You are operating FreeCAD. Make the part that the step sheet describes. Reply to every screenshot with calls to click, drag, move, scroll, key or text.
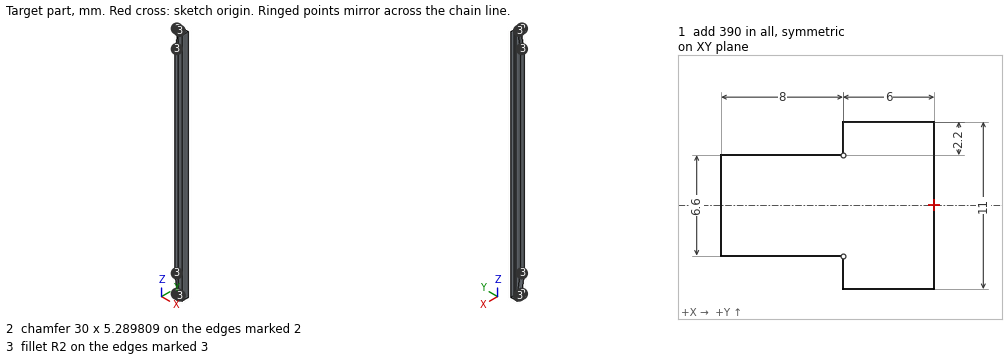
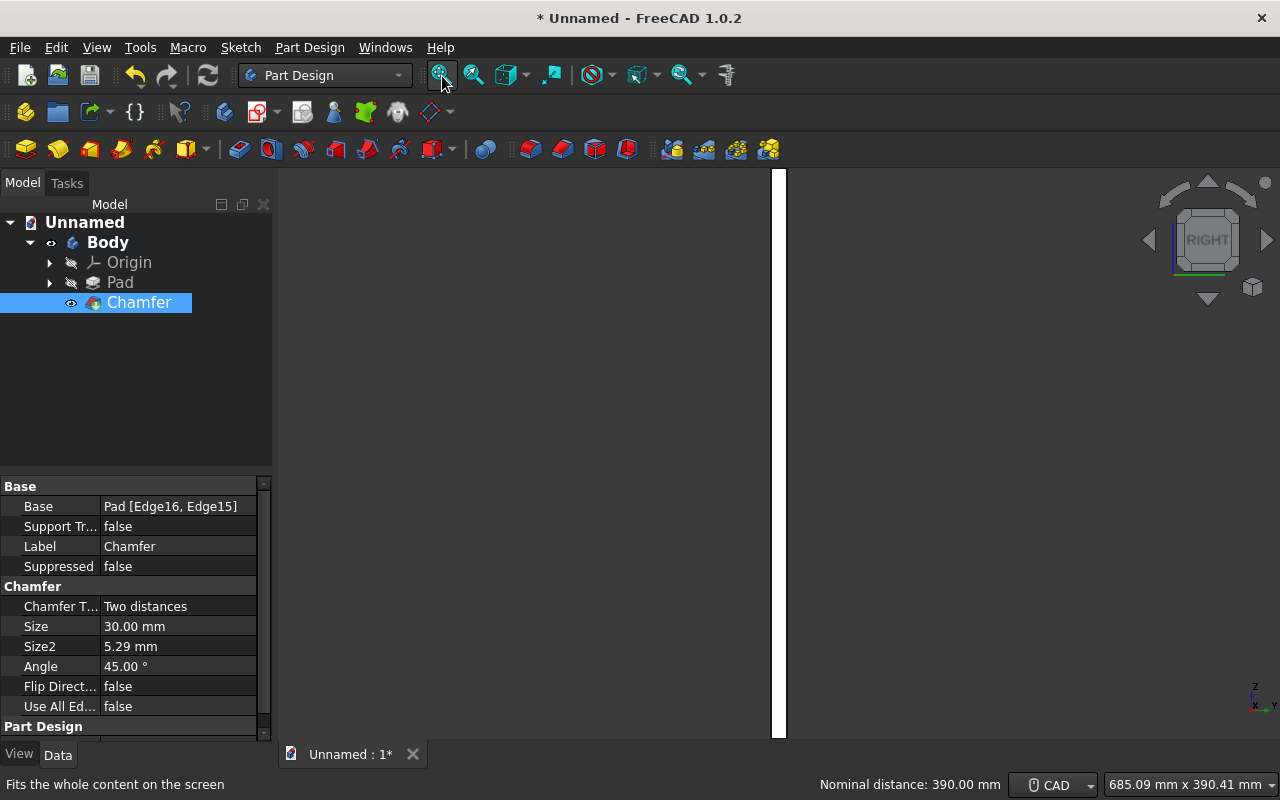
click(442, 76)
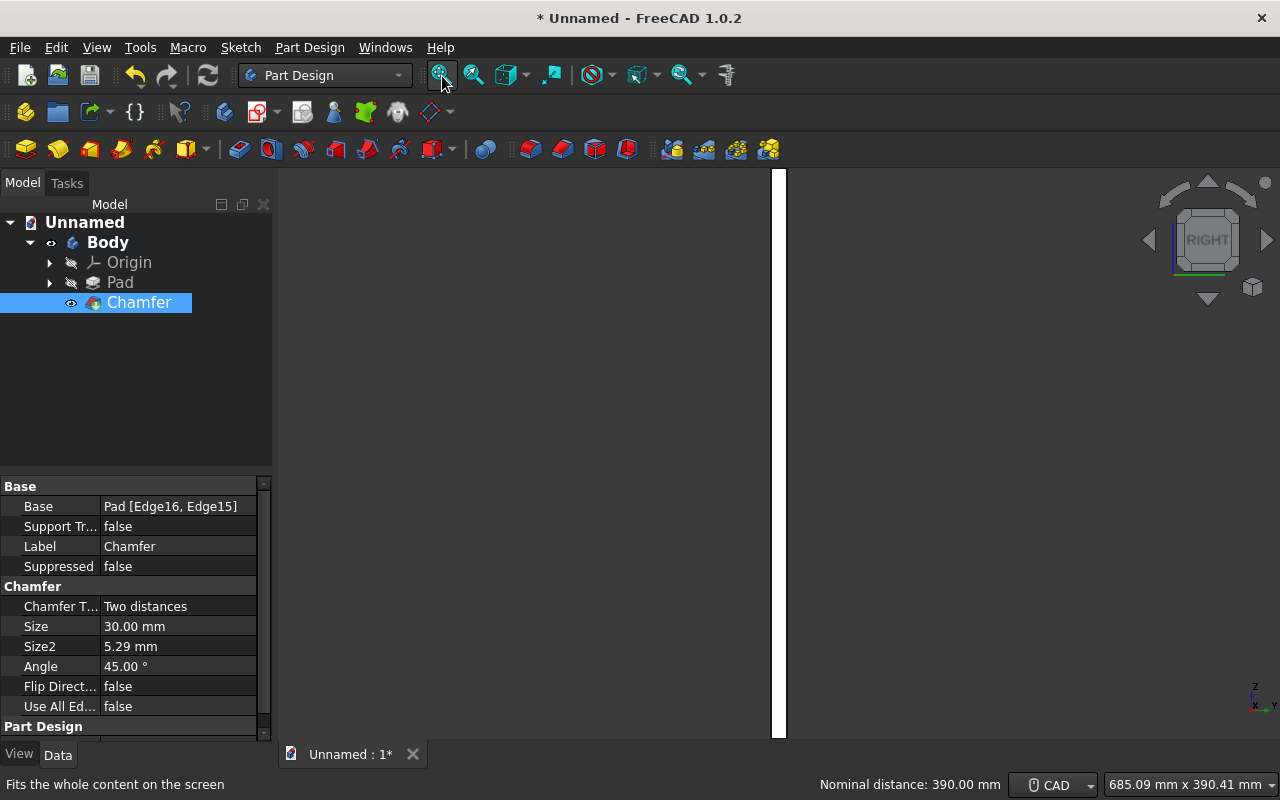
scroll(779, 211, up, 8)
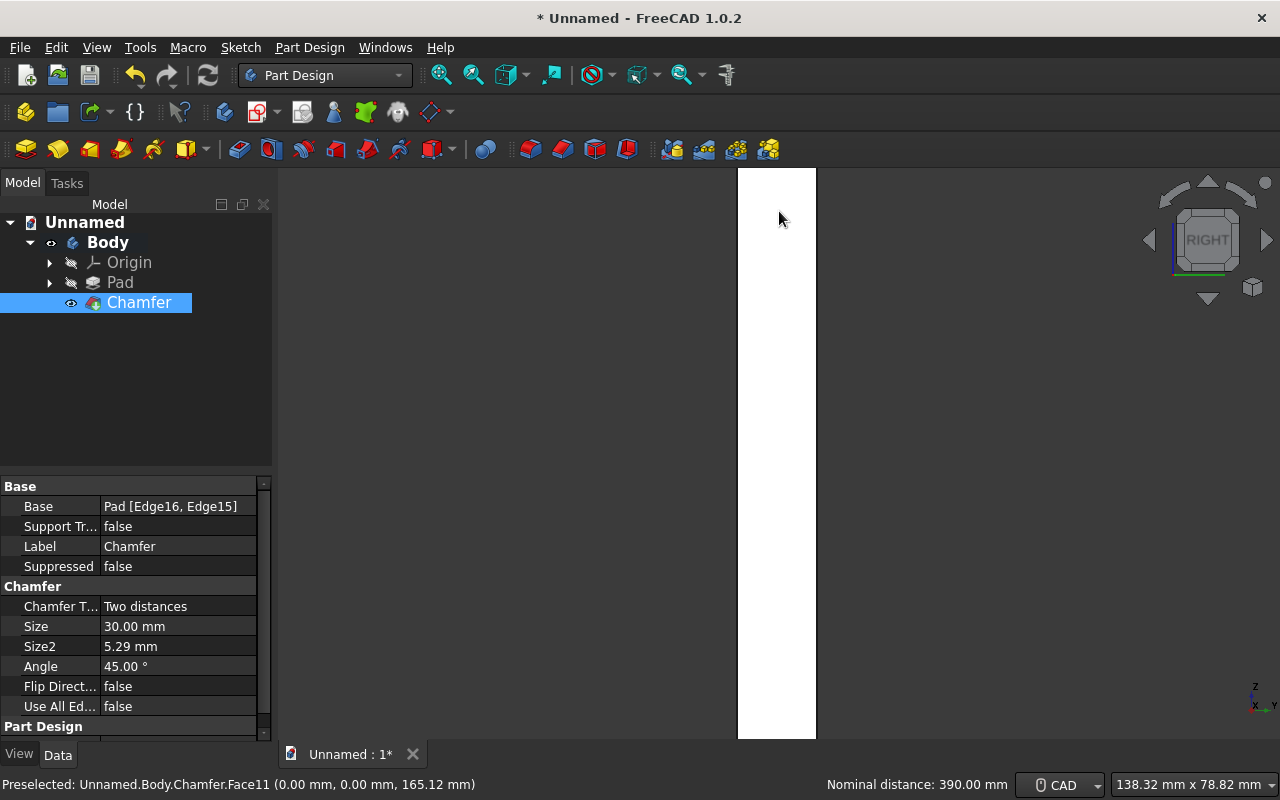
click(442, 76)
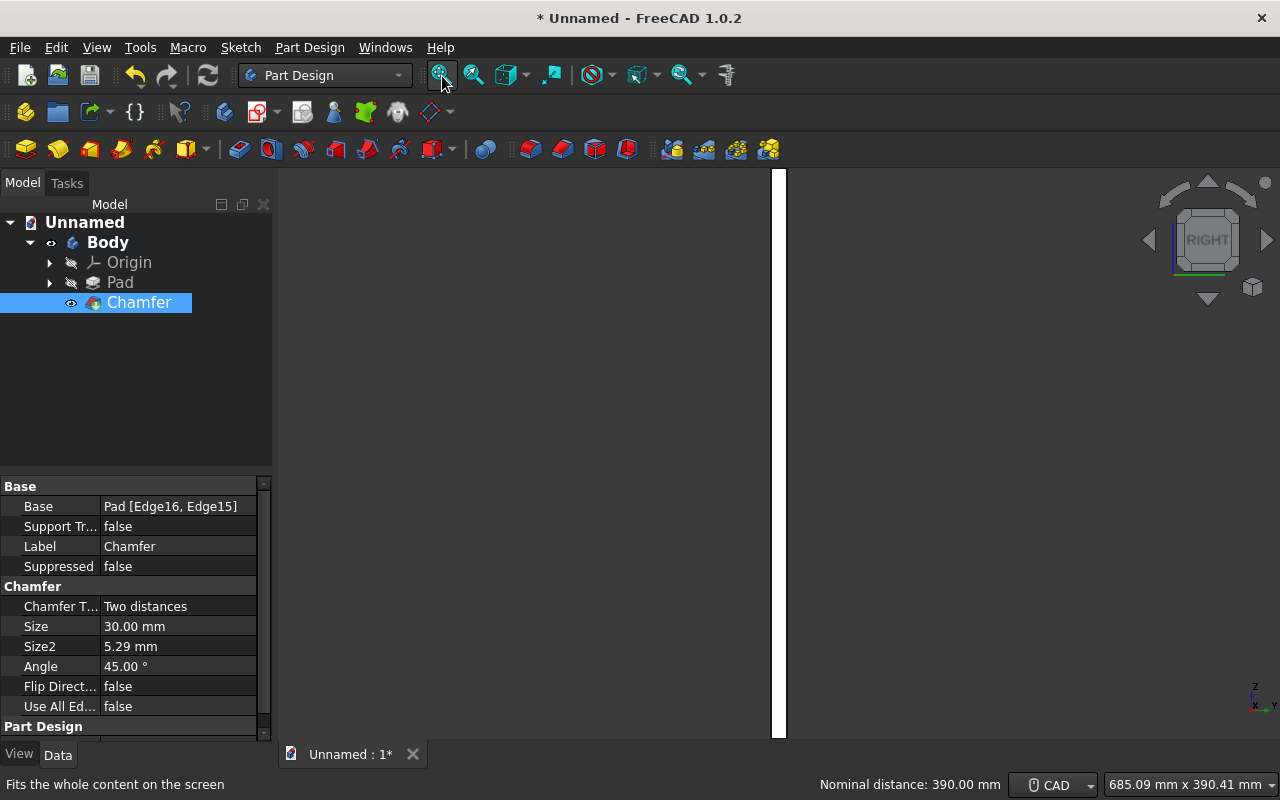
key(5)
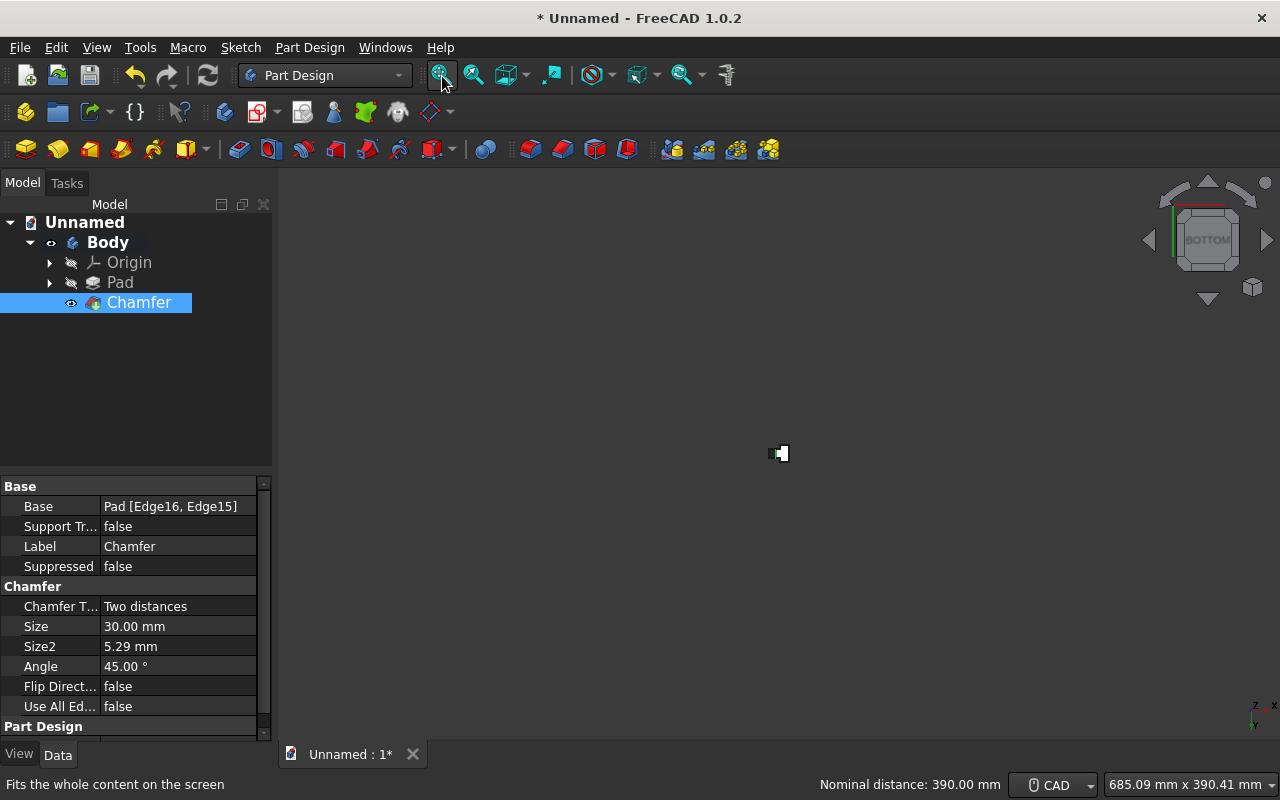
click(442, 76)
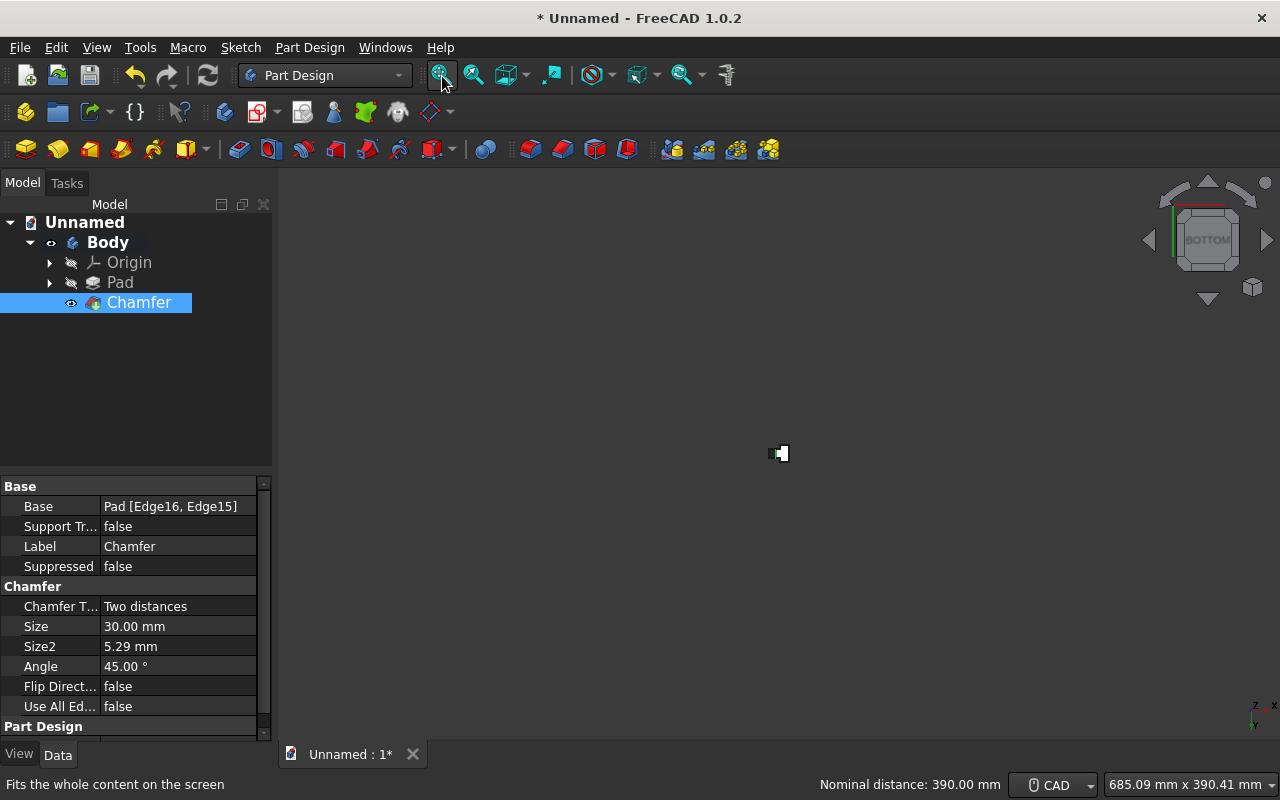
scroll(769, 452, up, 8)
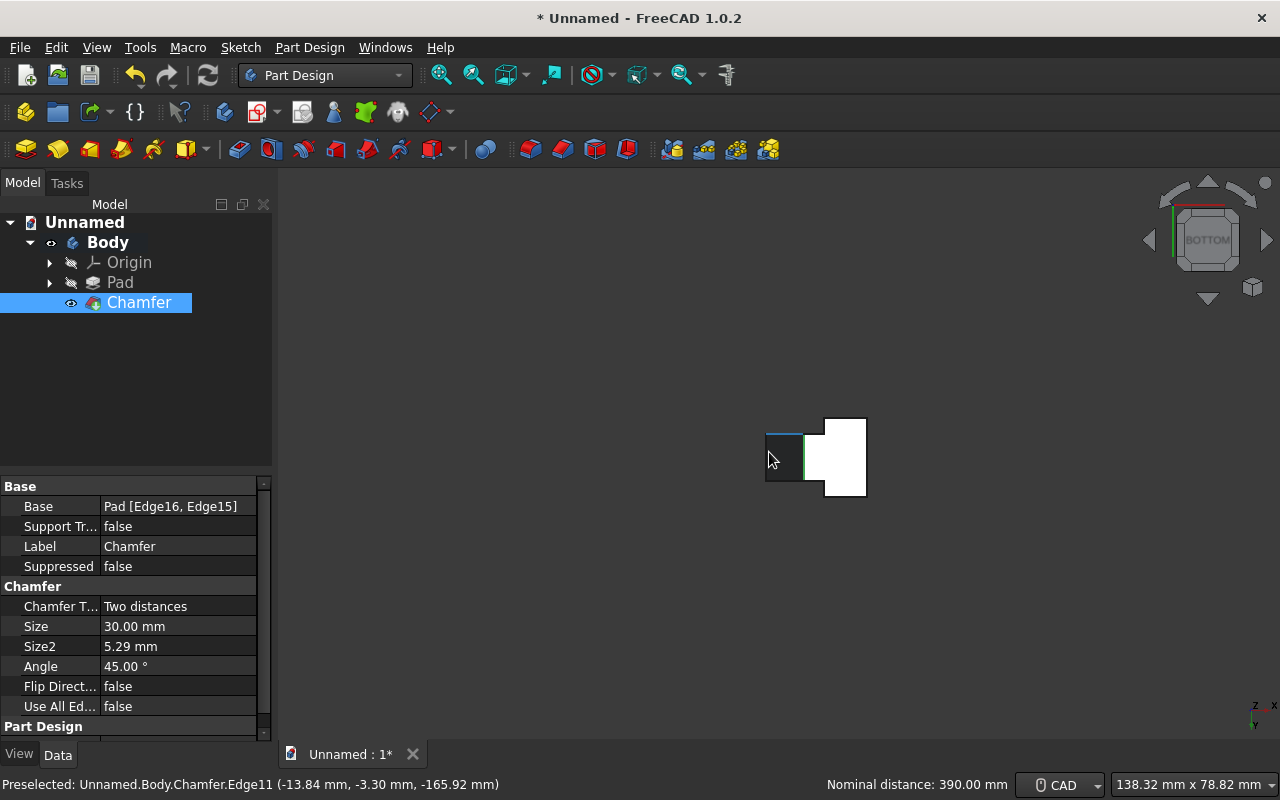
click(442, 76)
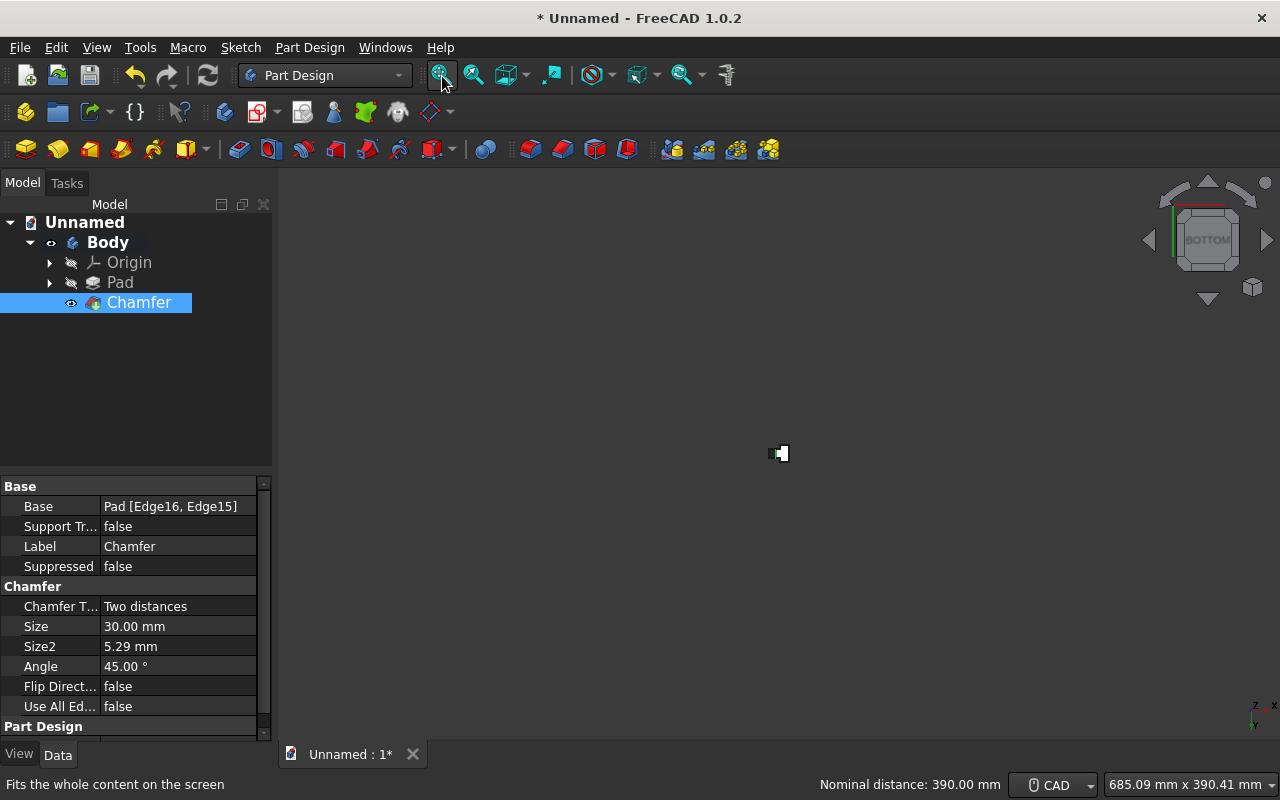
key(4)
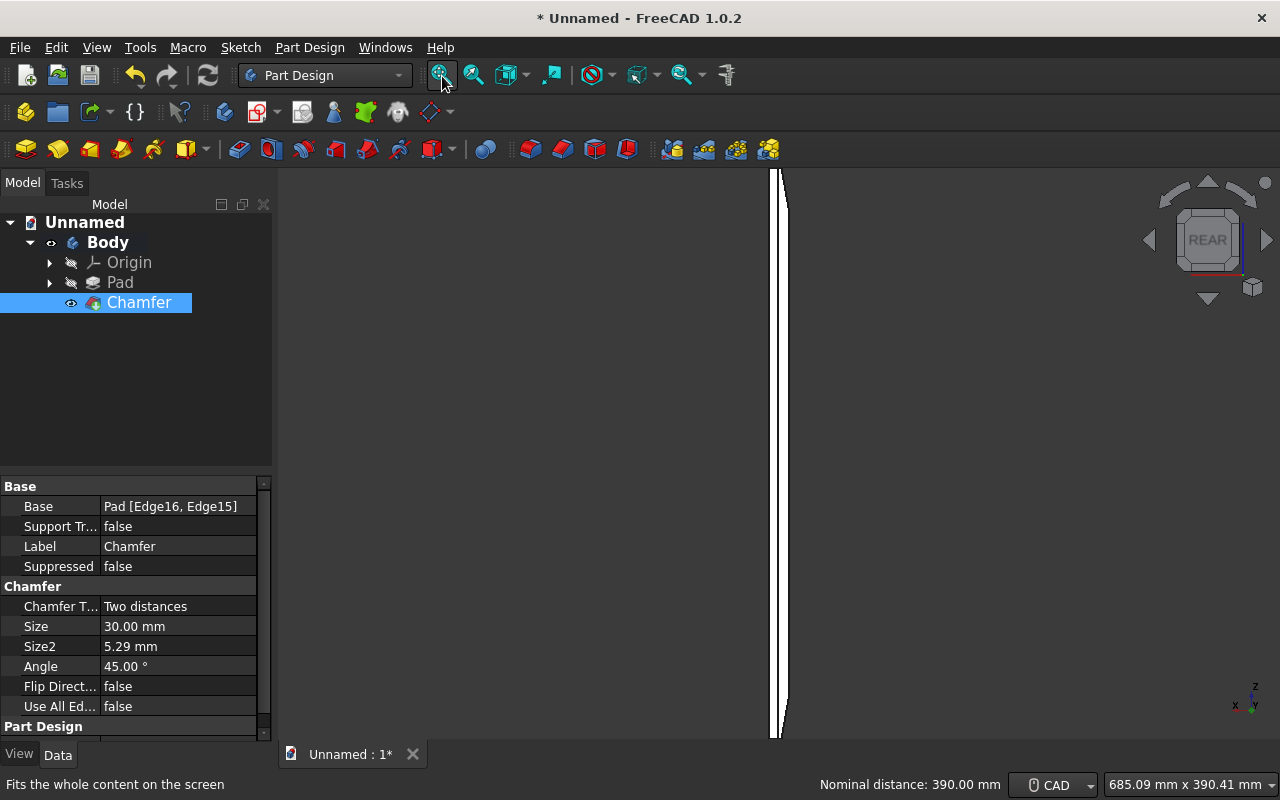
click(442, 76)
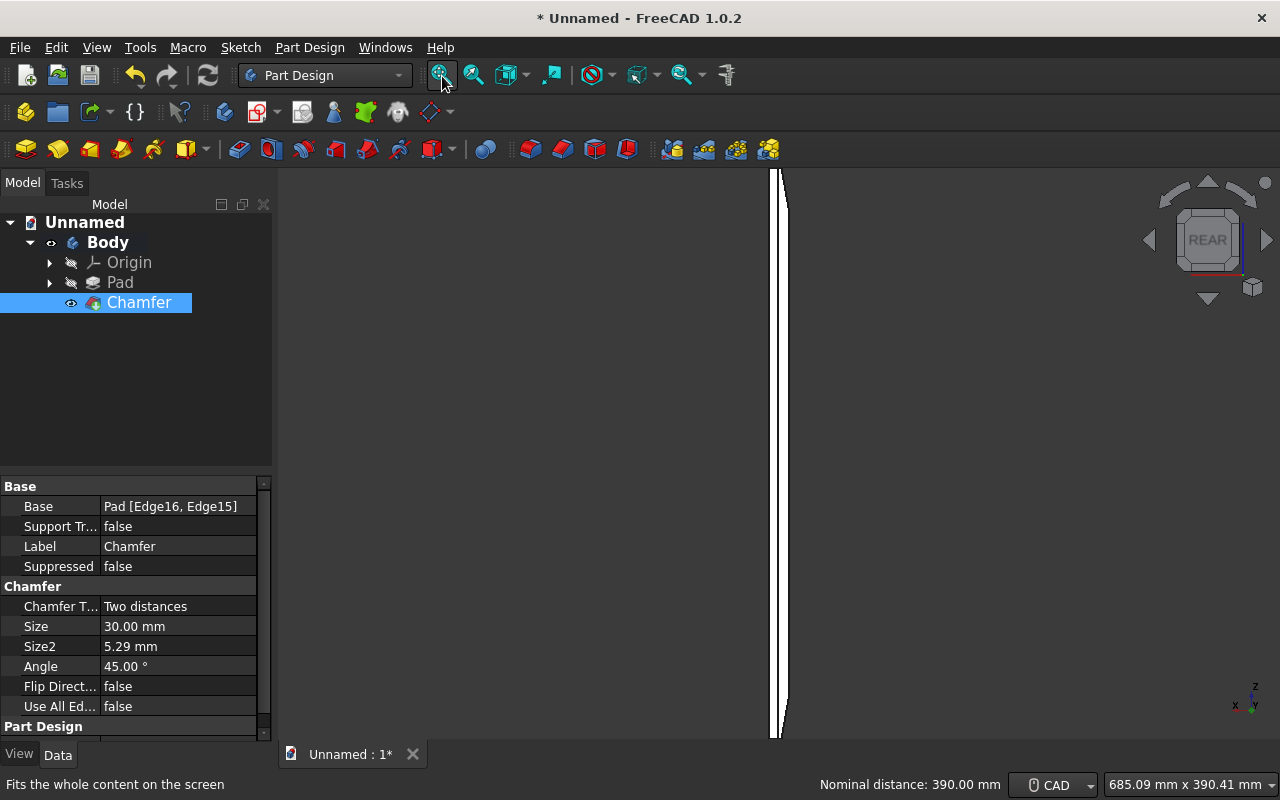
scroll(789, 211, up, 8)